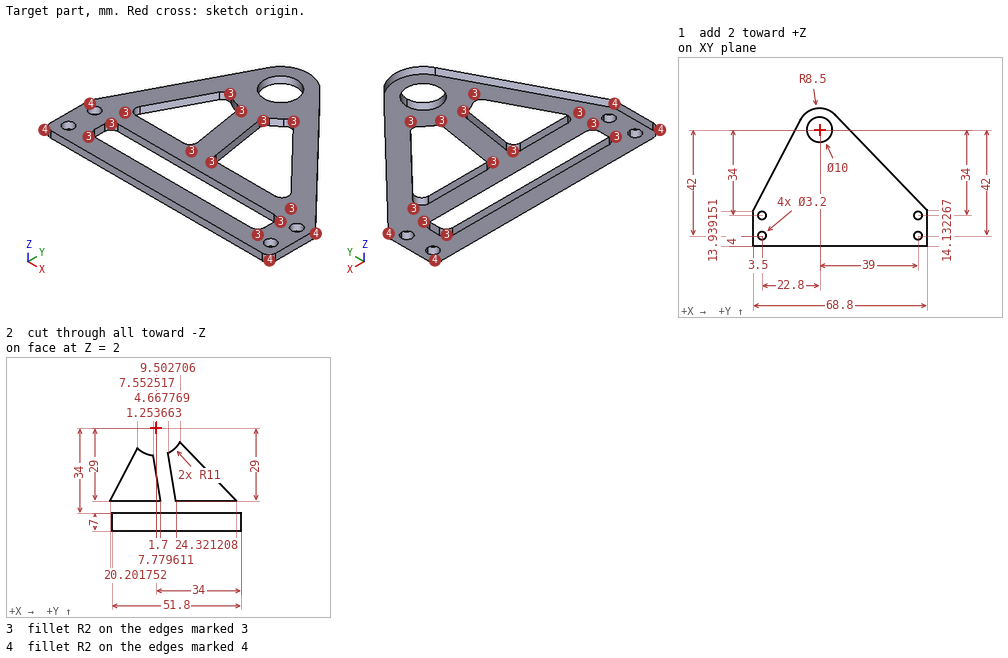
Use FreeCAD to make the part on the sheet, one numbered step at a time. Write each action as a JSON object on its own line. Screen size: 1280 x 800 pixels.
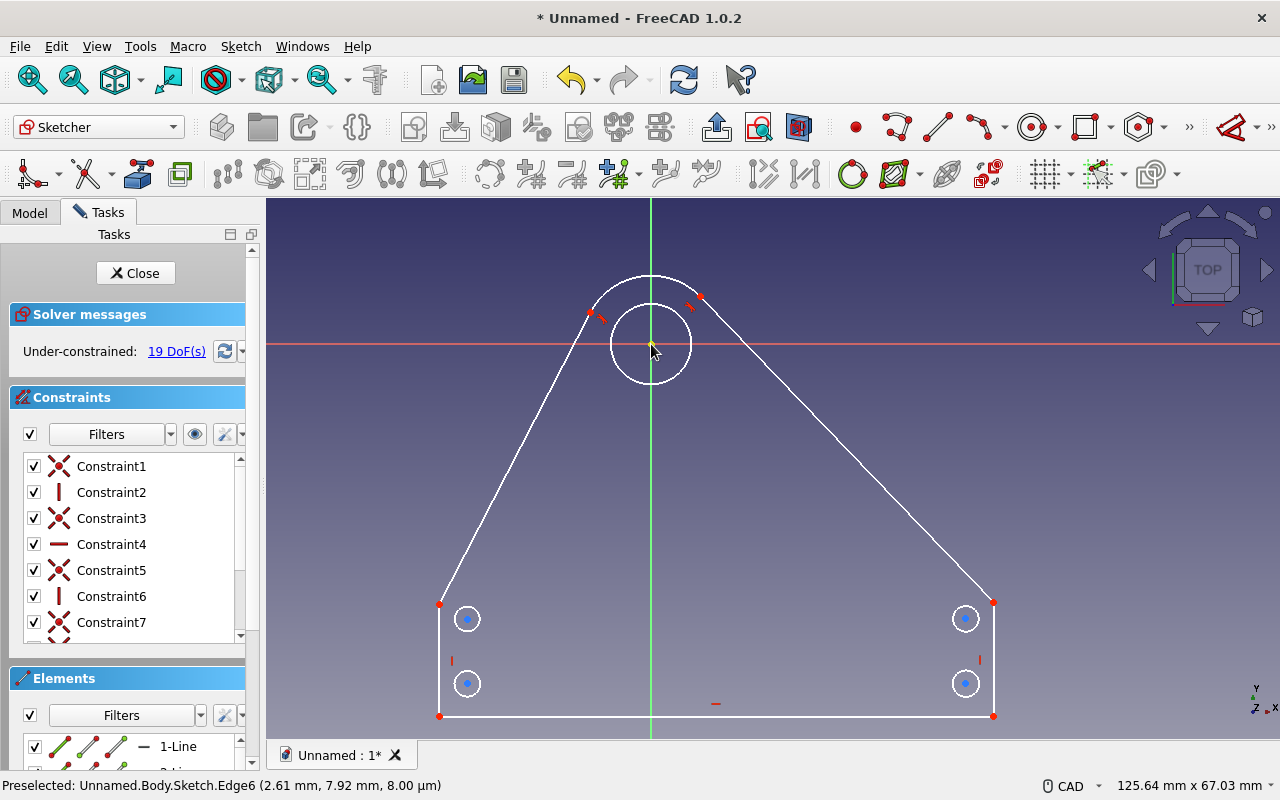
{"action": "scroll", "coordinate": [508, 615], "scroll_direction": "up", "scroll_amount": 2}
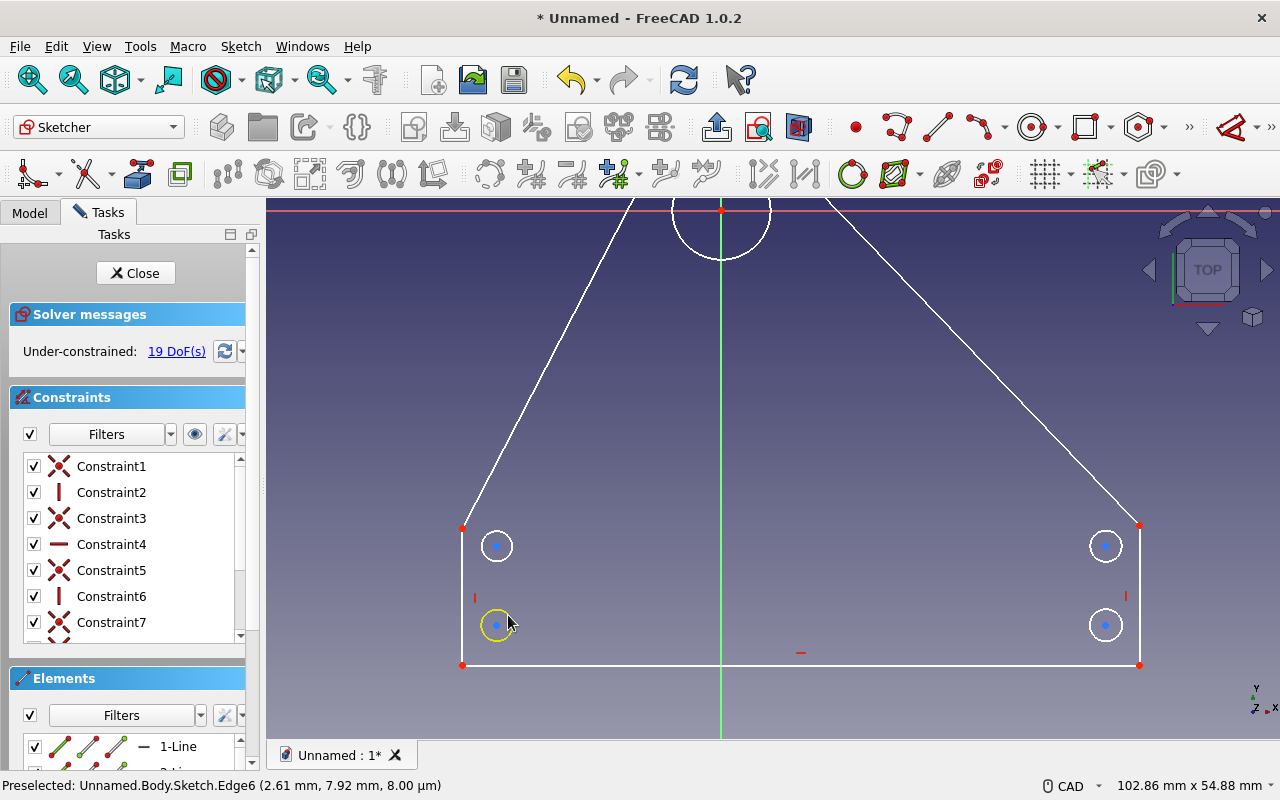
{"action": "left_click", "coordinate": [508, 614]}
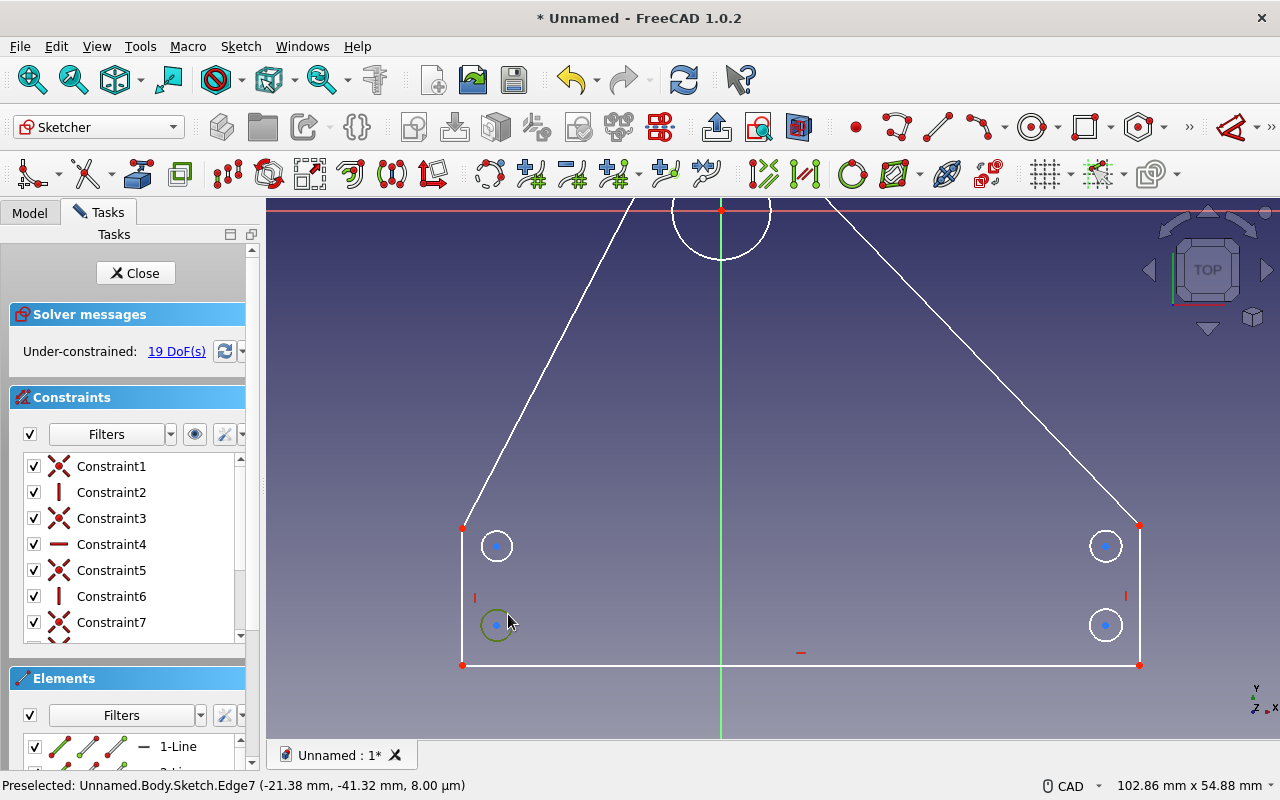
{"action": "left_click", "coordinate": [508, 536]}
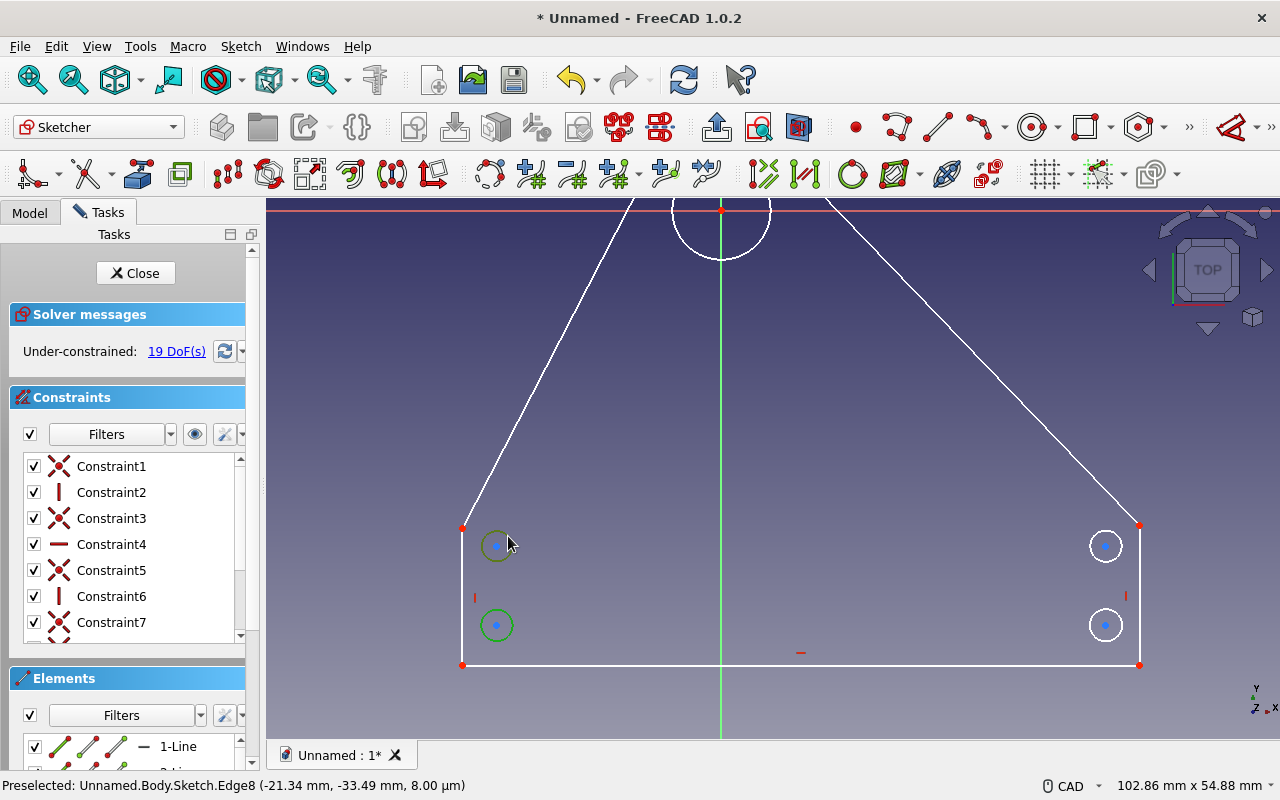
{"action": "left_click", "coordinate": [1095, 614]}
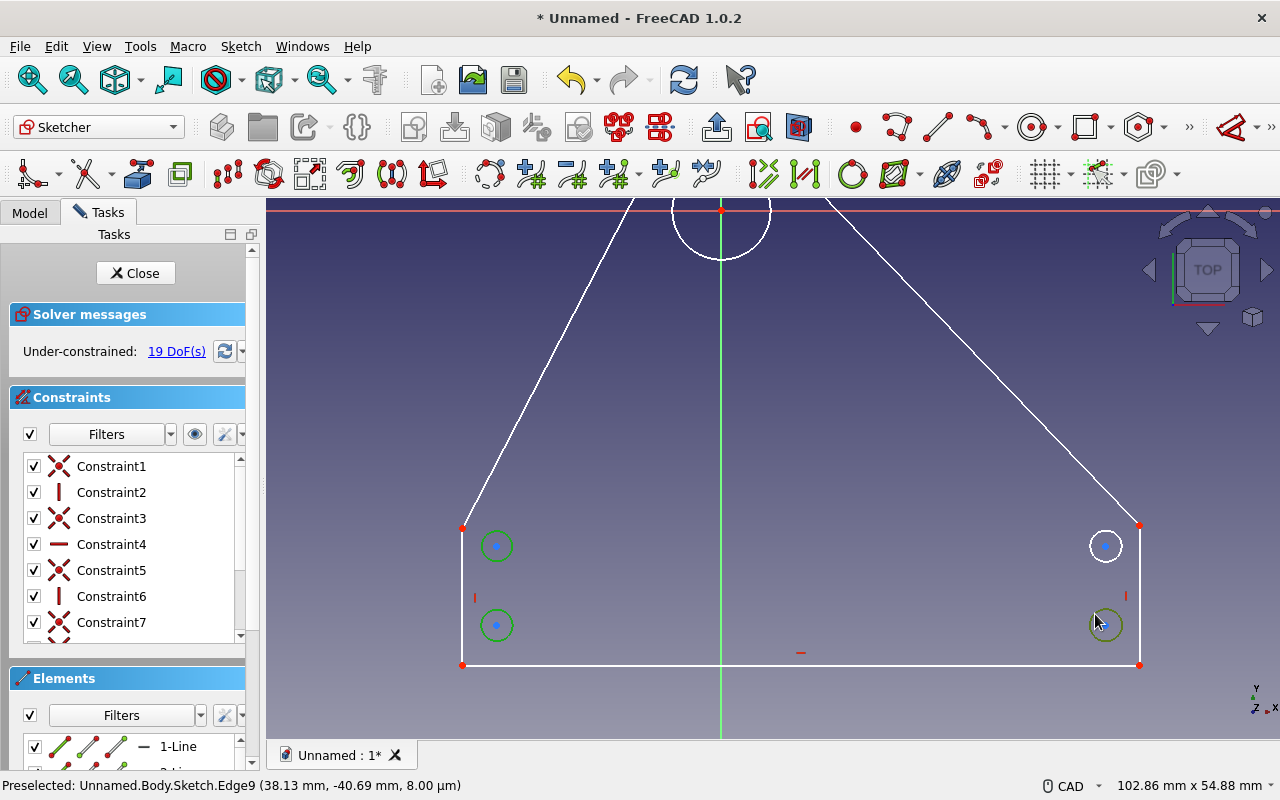
{"action": "left_click", "coordinate": [1095, 535]}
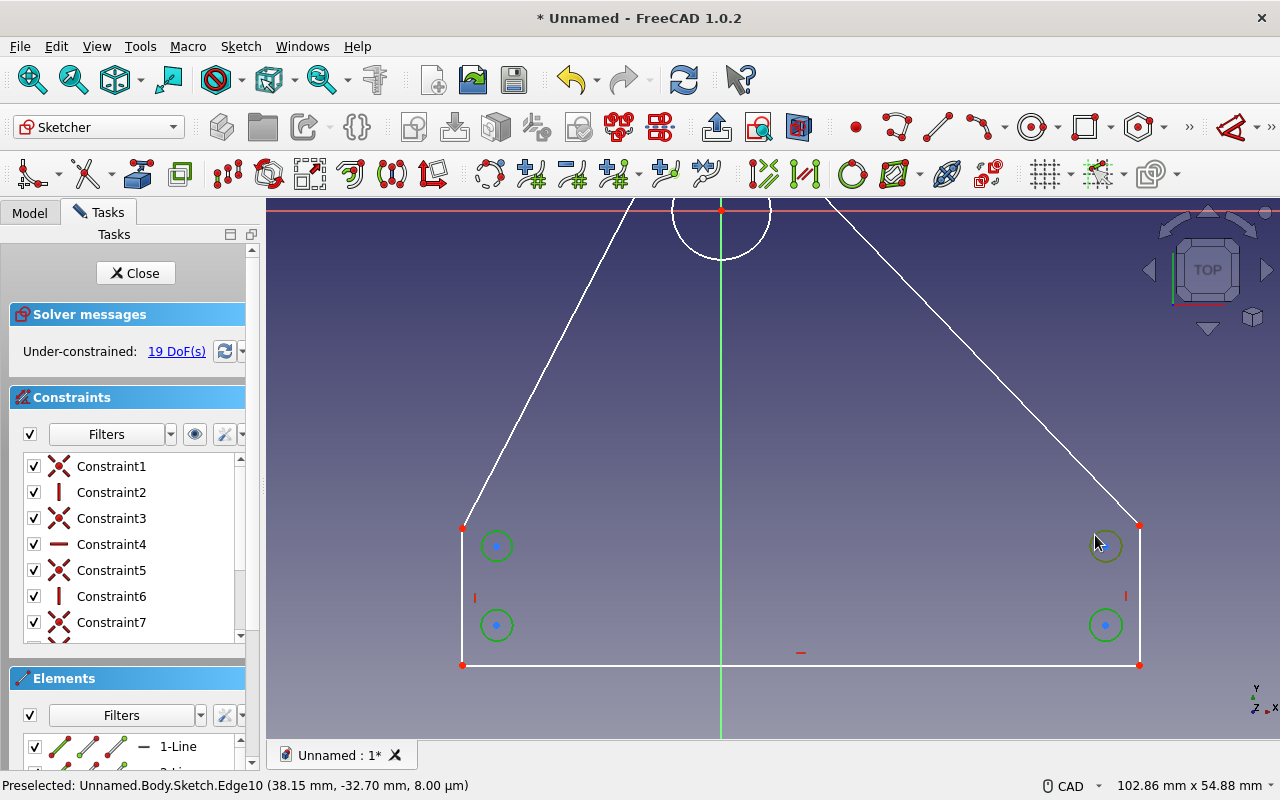
{"action": "key", "text": "e"}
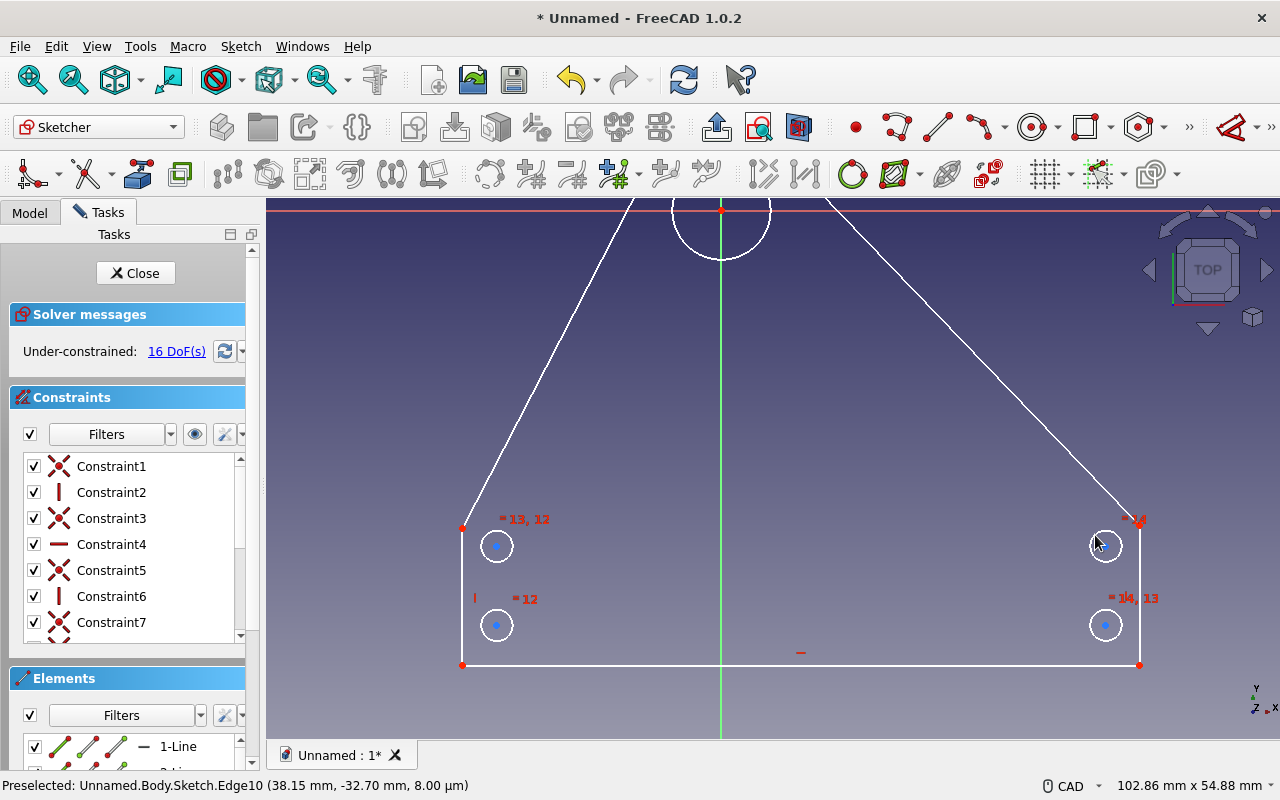
{"action": "left_click", "coordinate": [497, 625]}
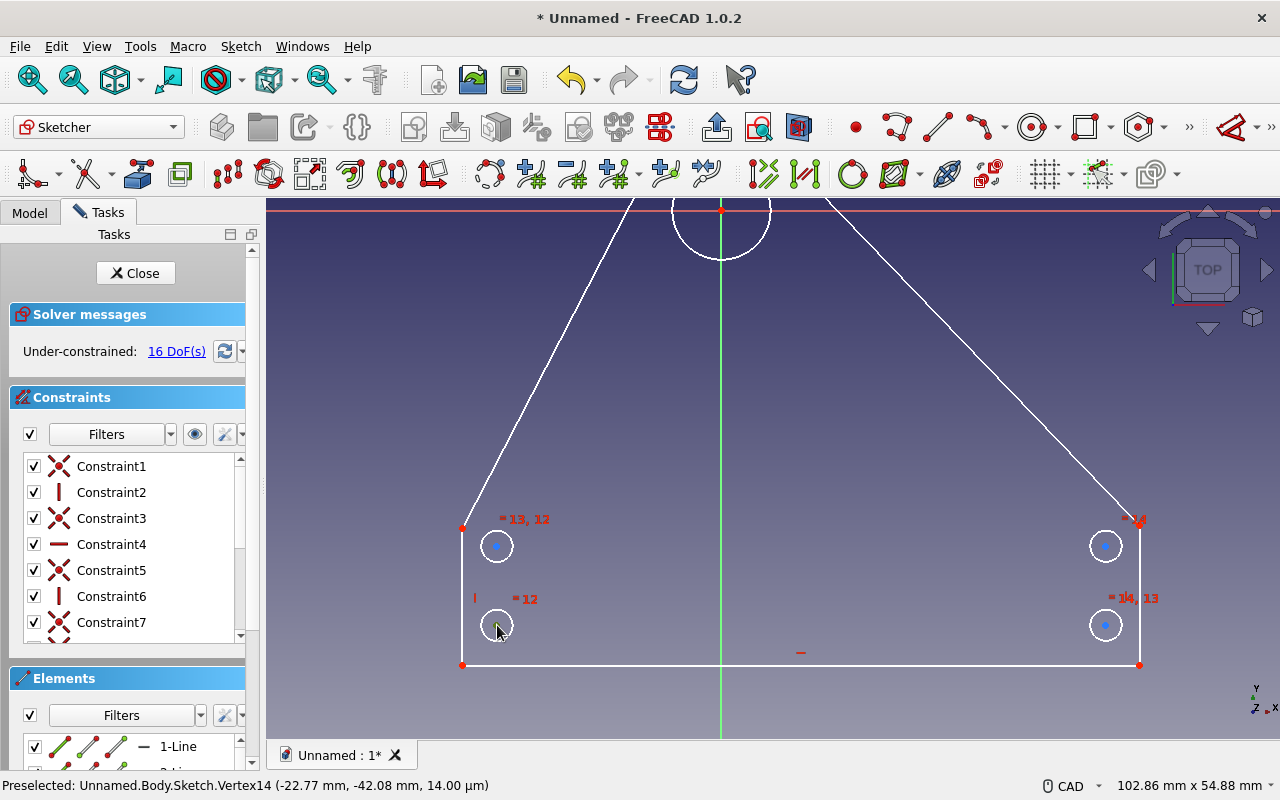
{"action": "left_click", "coordinate": [497, 546]}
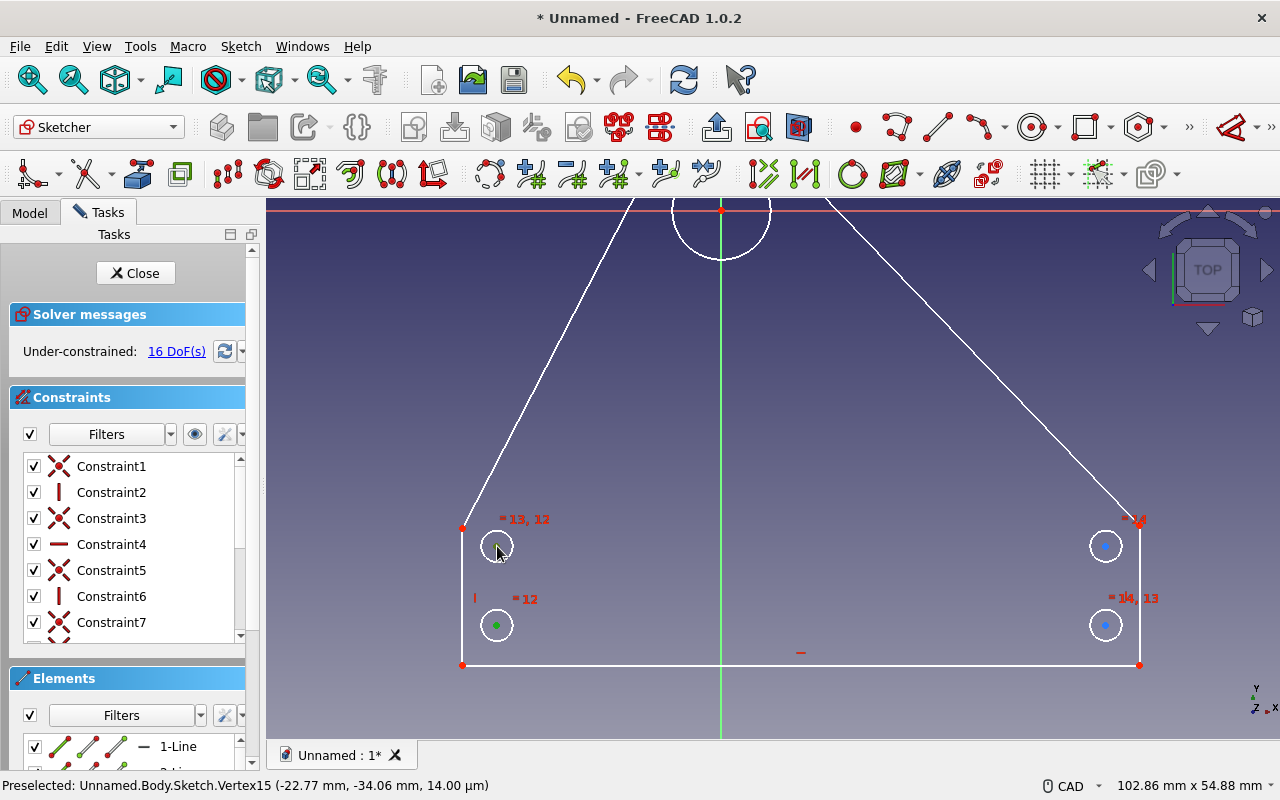
{"action": "key", "text": "v"}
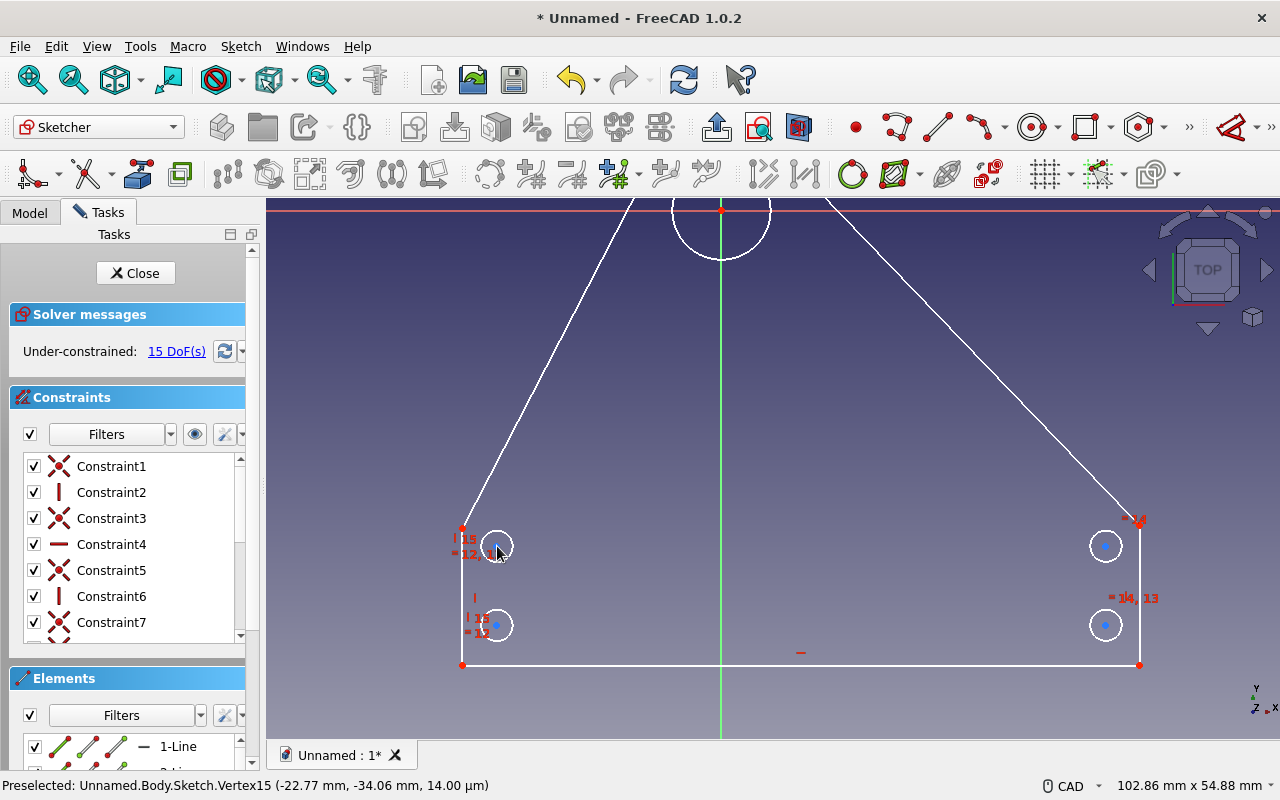
{"action": "left_click", "coordinate": [1106, 625]}